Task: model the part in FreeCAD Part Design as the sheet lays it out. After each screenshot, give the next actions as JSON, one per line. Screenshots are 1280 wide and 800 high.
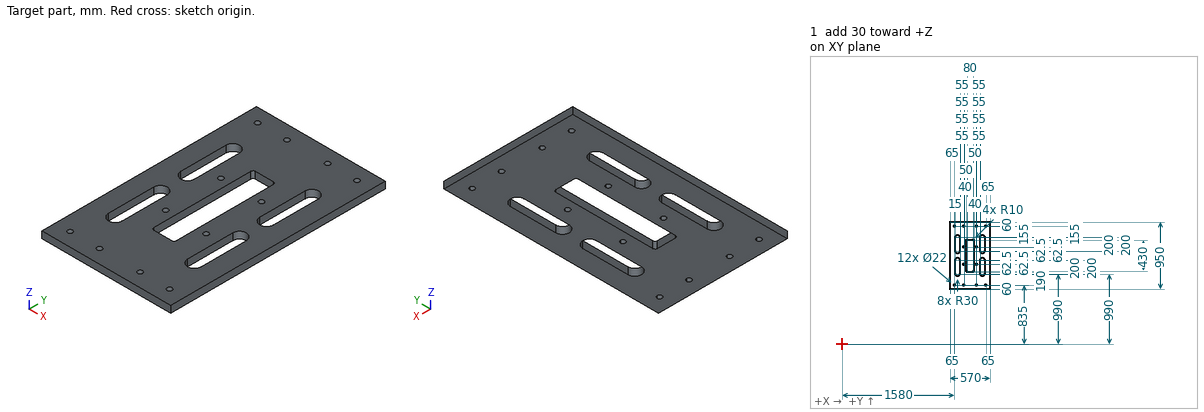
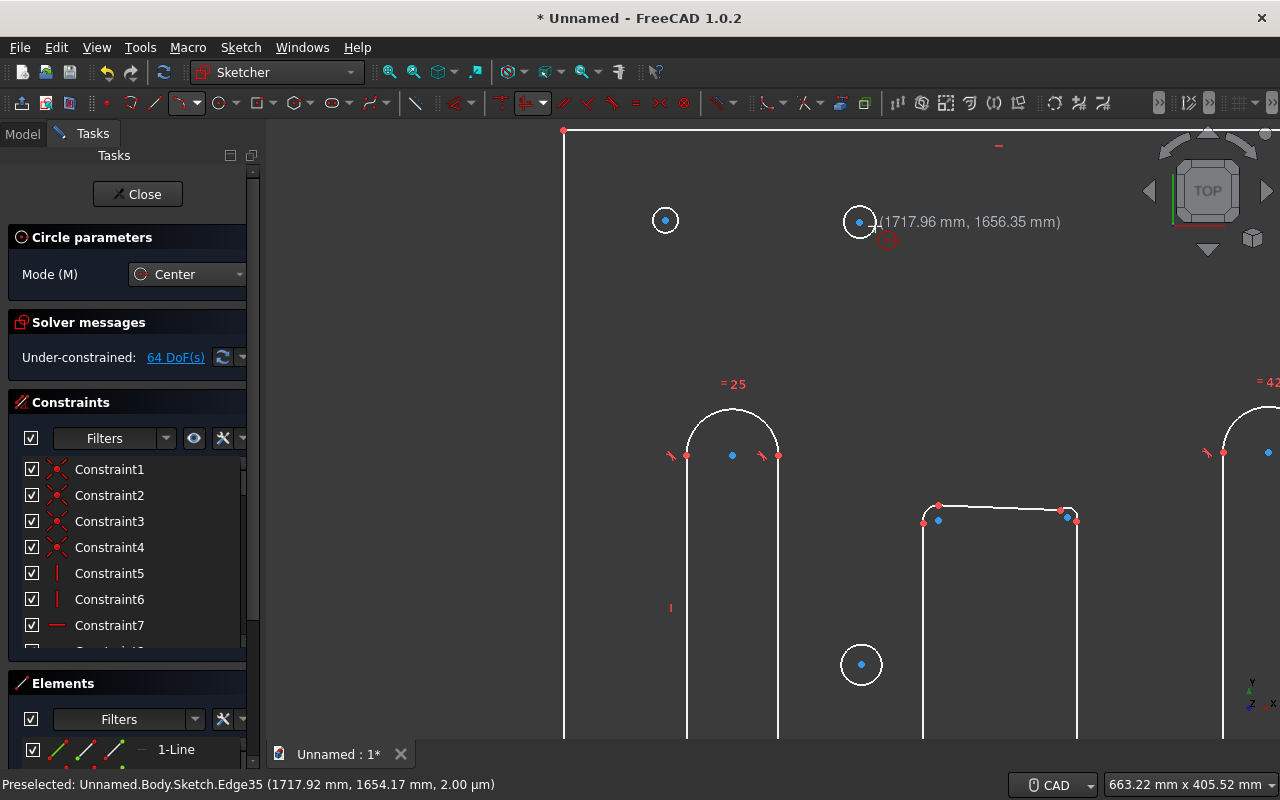
{"action": "scroll", "coordinate": [875, 229], "scroll_direction": "down", "scroll_amount": 9}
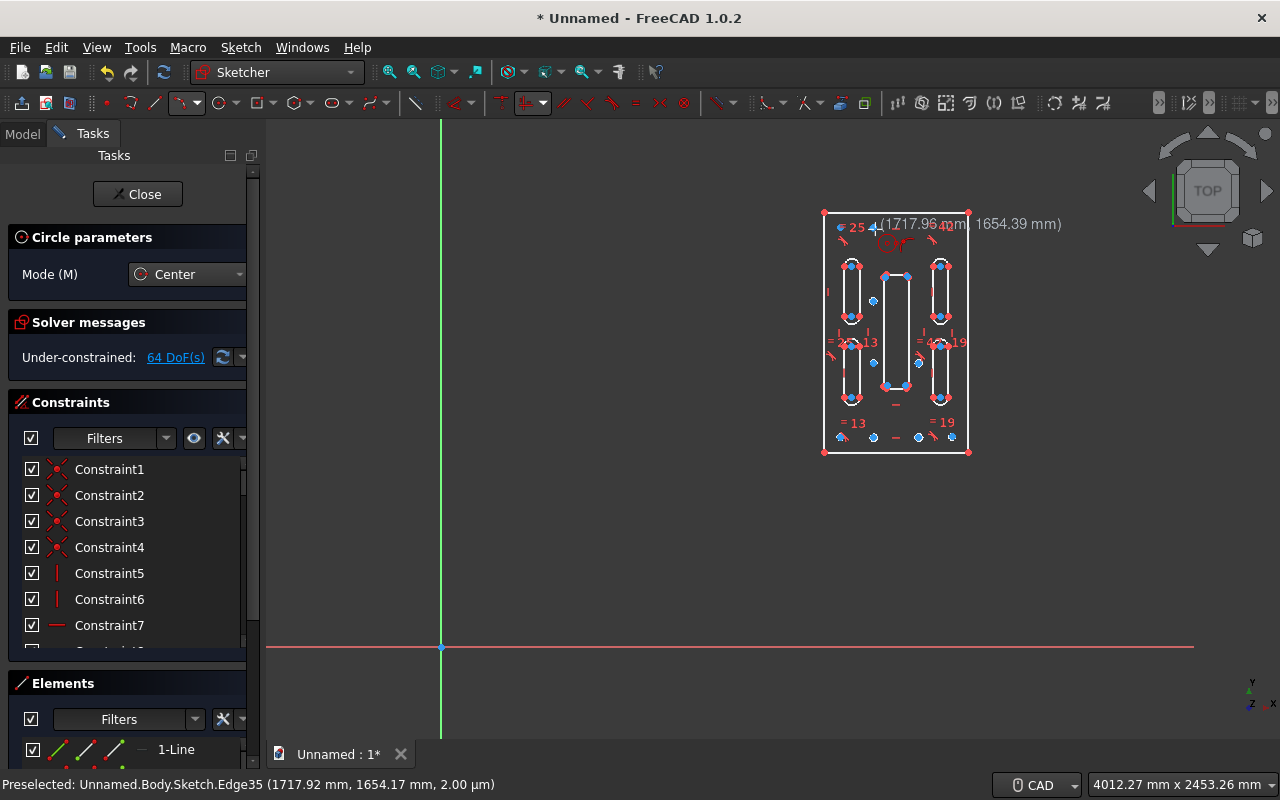
{"action": "scroll", "coordinate": [919, 301], "scroll_direction": "up", "scroll_amount": 11}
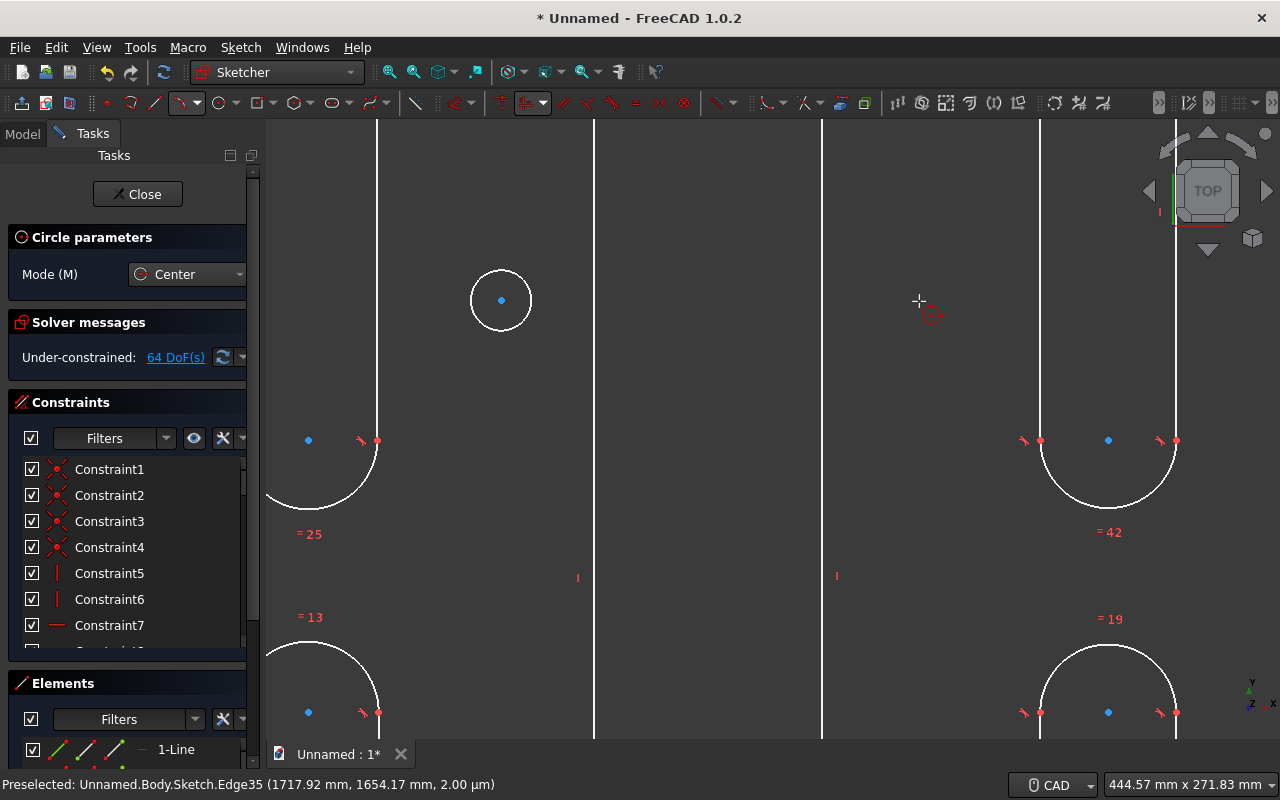
{"action": "scroll", "coordinate": [919, 301], "scroll_direction": "down", "scroll_amount": 11}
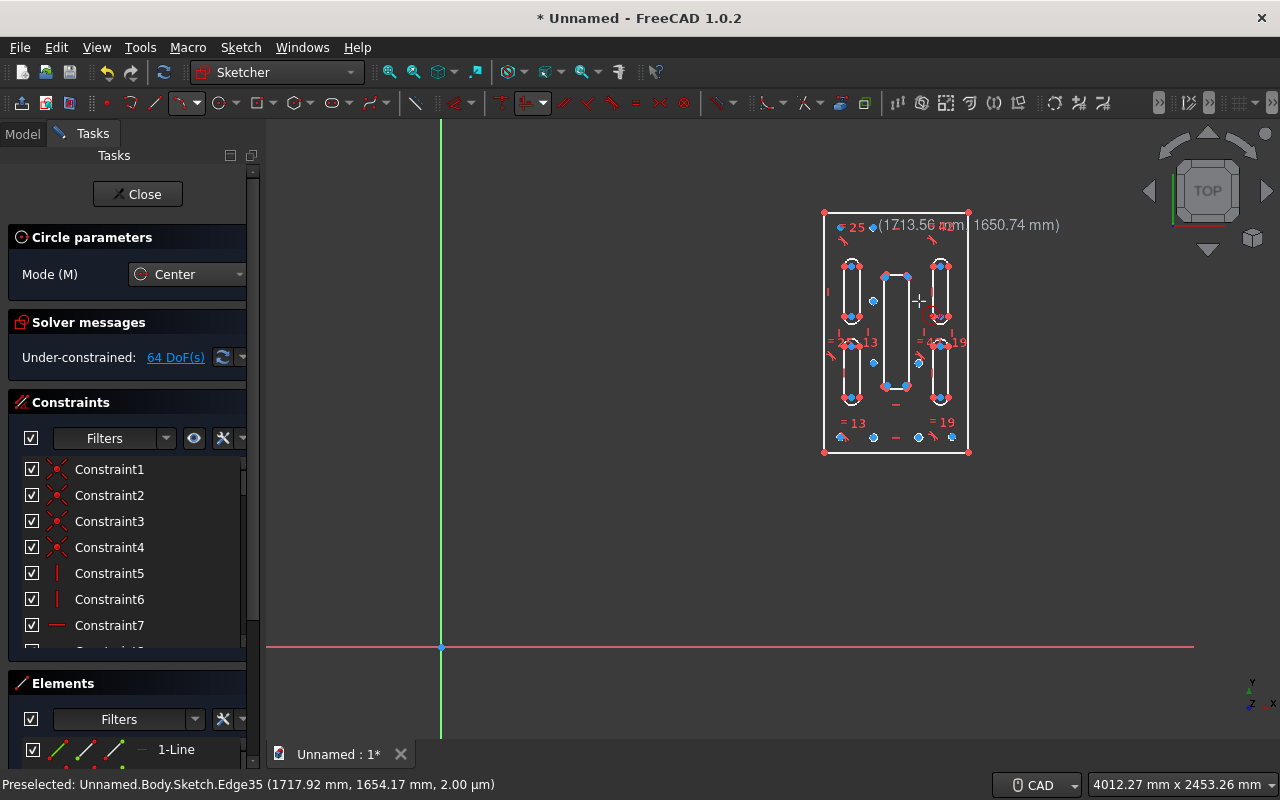
{"action": "scroll", "coordinate": [919, 301], "scroll_direction": "up", "scroll_amount": 3}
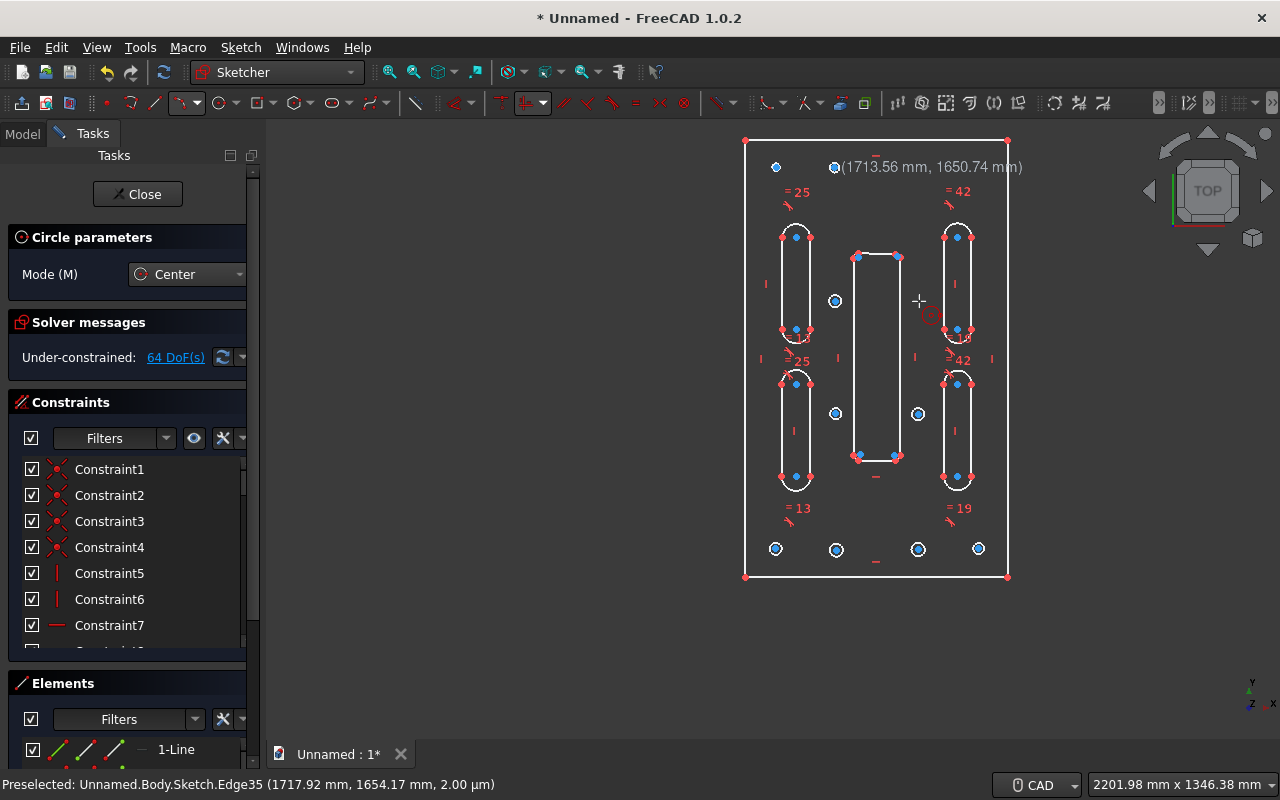
{"action": "left_click", "coordinate": [918, 300]}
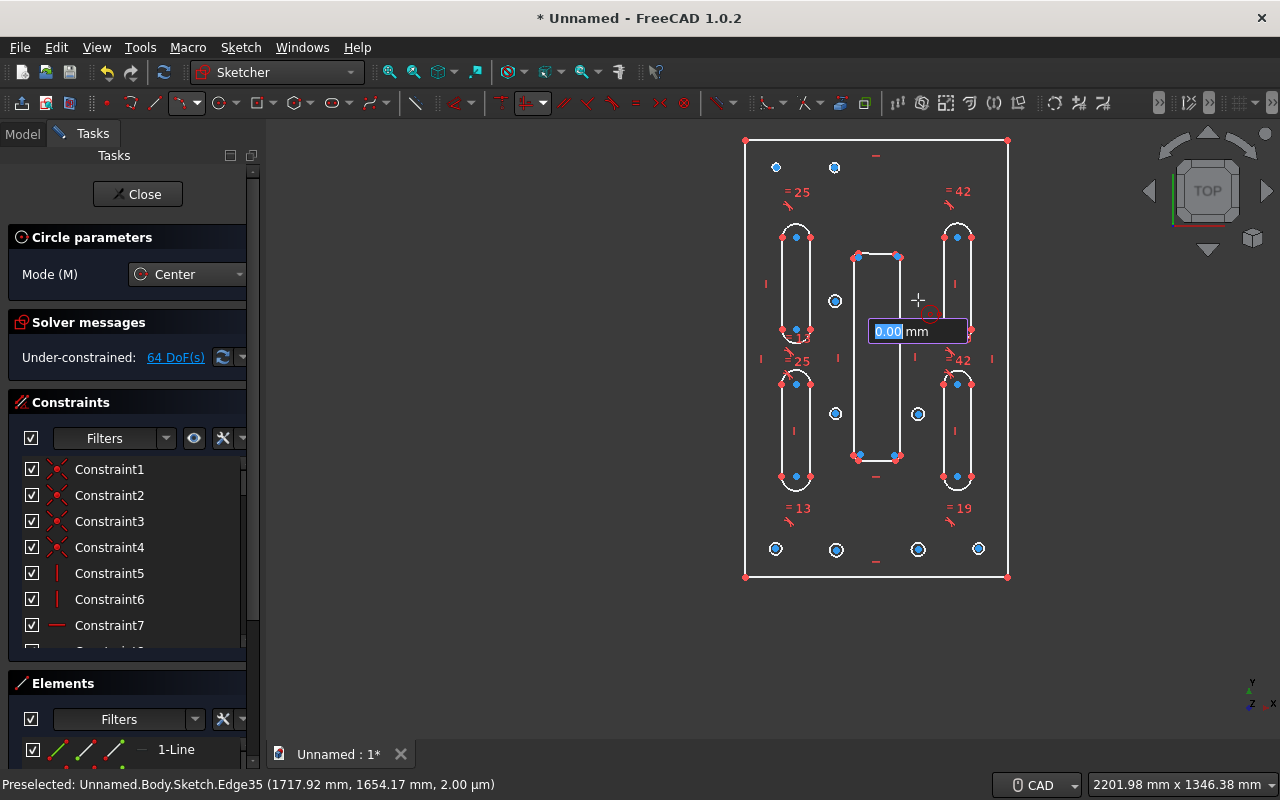
{"action": "scroll", "coordinate": [922, 296], "scroll_direction": "up", "scroll_amount": 6}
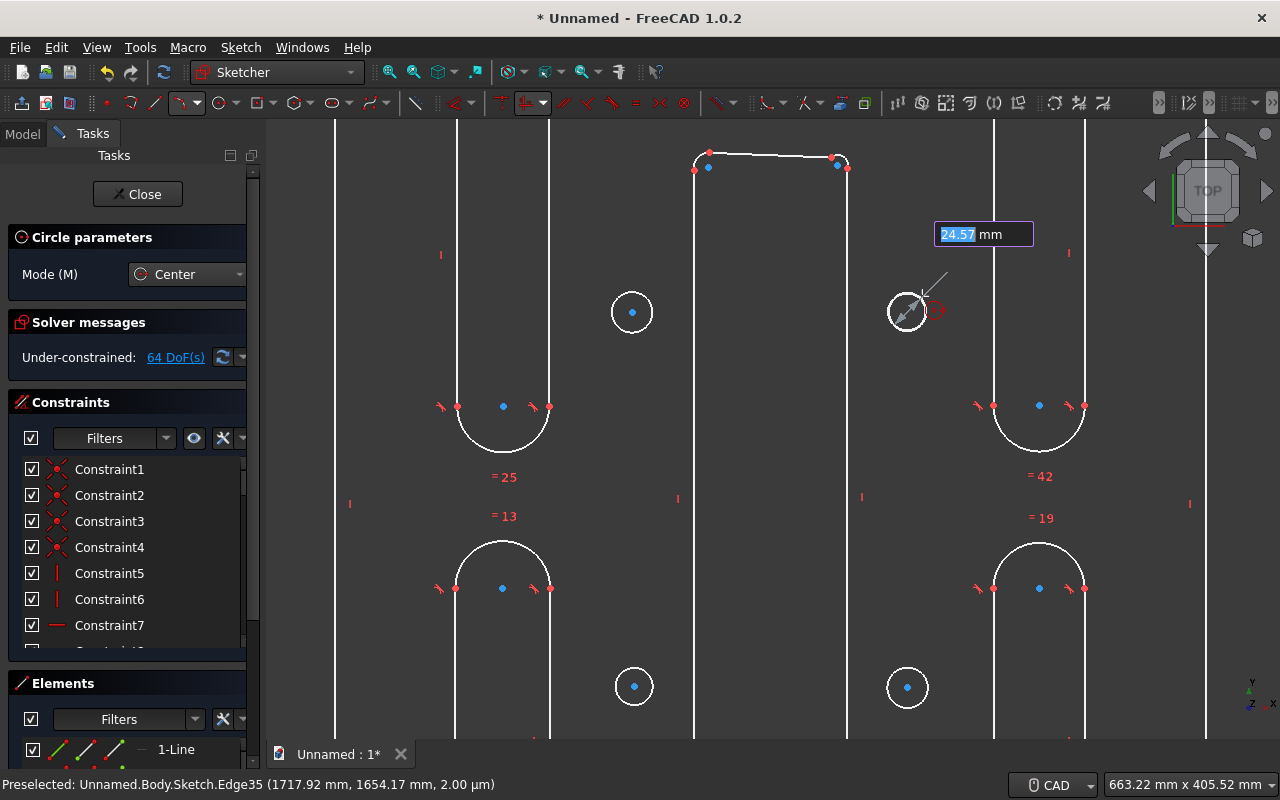
{"action": "left_click", "coordinate": [921, 297]}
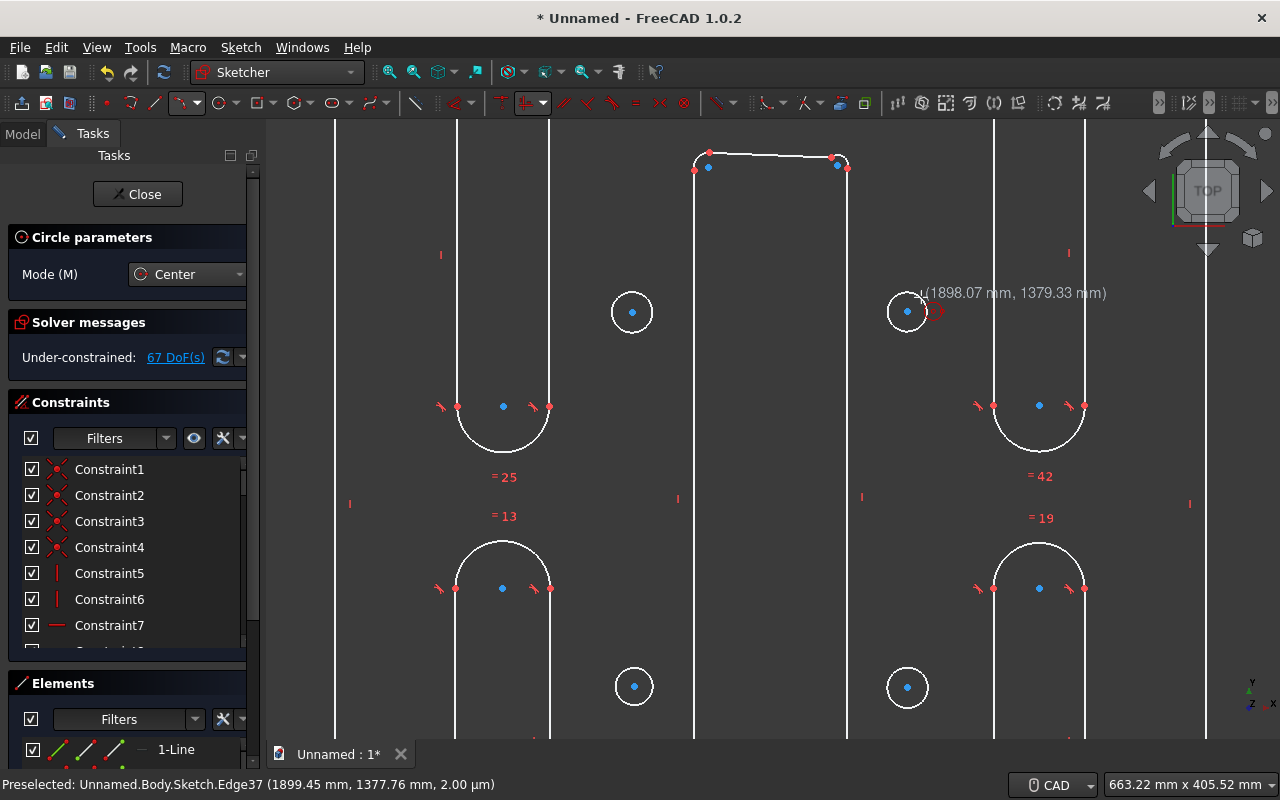
{"action": "scroll", "coordinate": [921, 298], "scroll_direction": "down", "scroll_amount": 9}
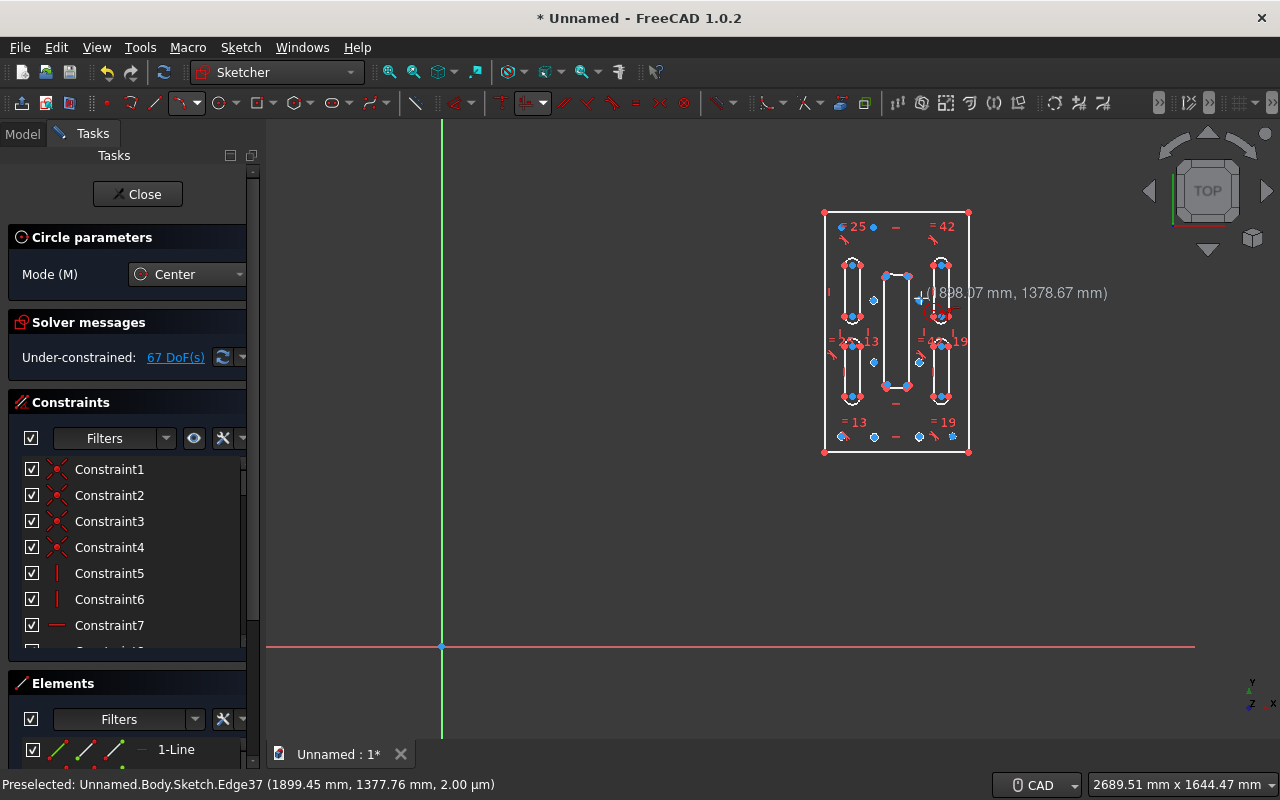
{"action": "scroll", "coordinate": [919, 226], "scroll_direction": "up", "scroll_amount": 11}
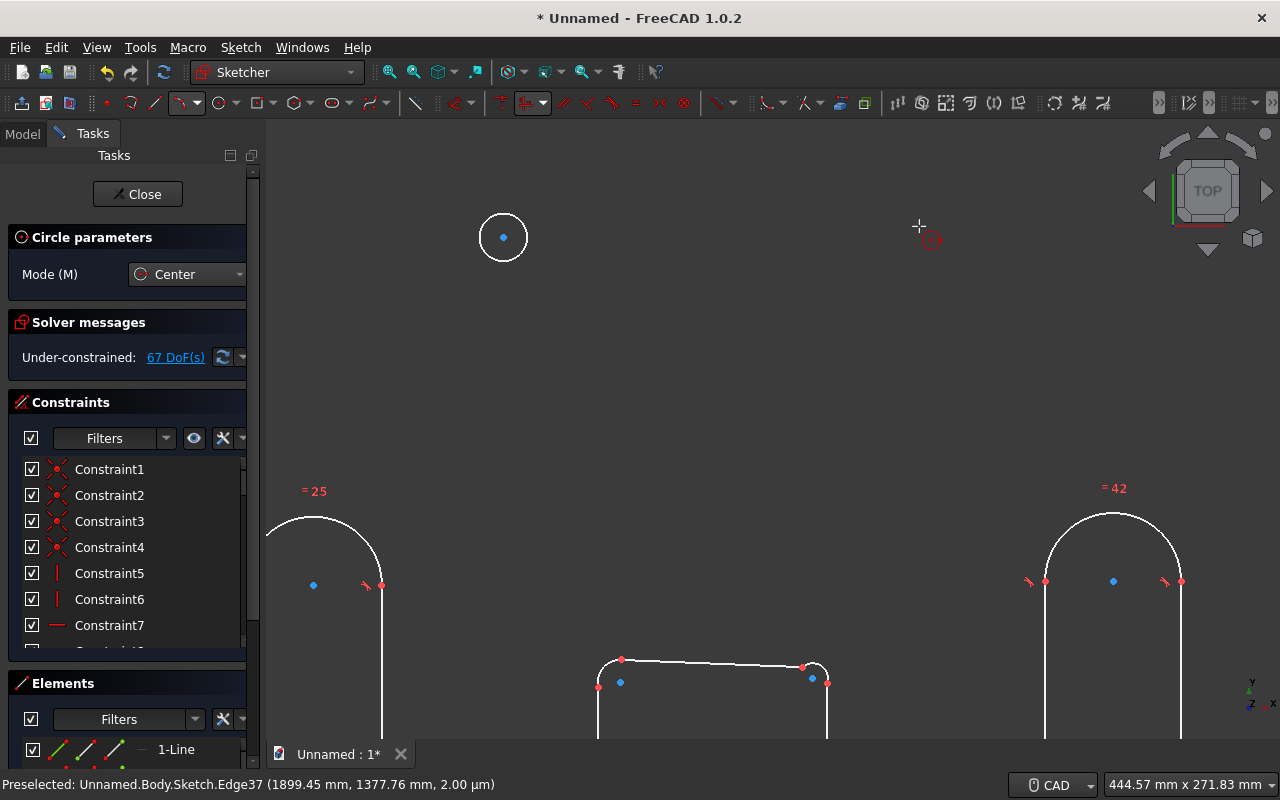
{"action": "scroll", "coordinate": [919, 226], "scroll_direction": "down", "scroll_amount": 11}